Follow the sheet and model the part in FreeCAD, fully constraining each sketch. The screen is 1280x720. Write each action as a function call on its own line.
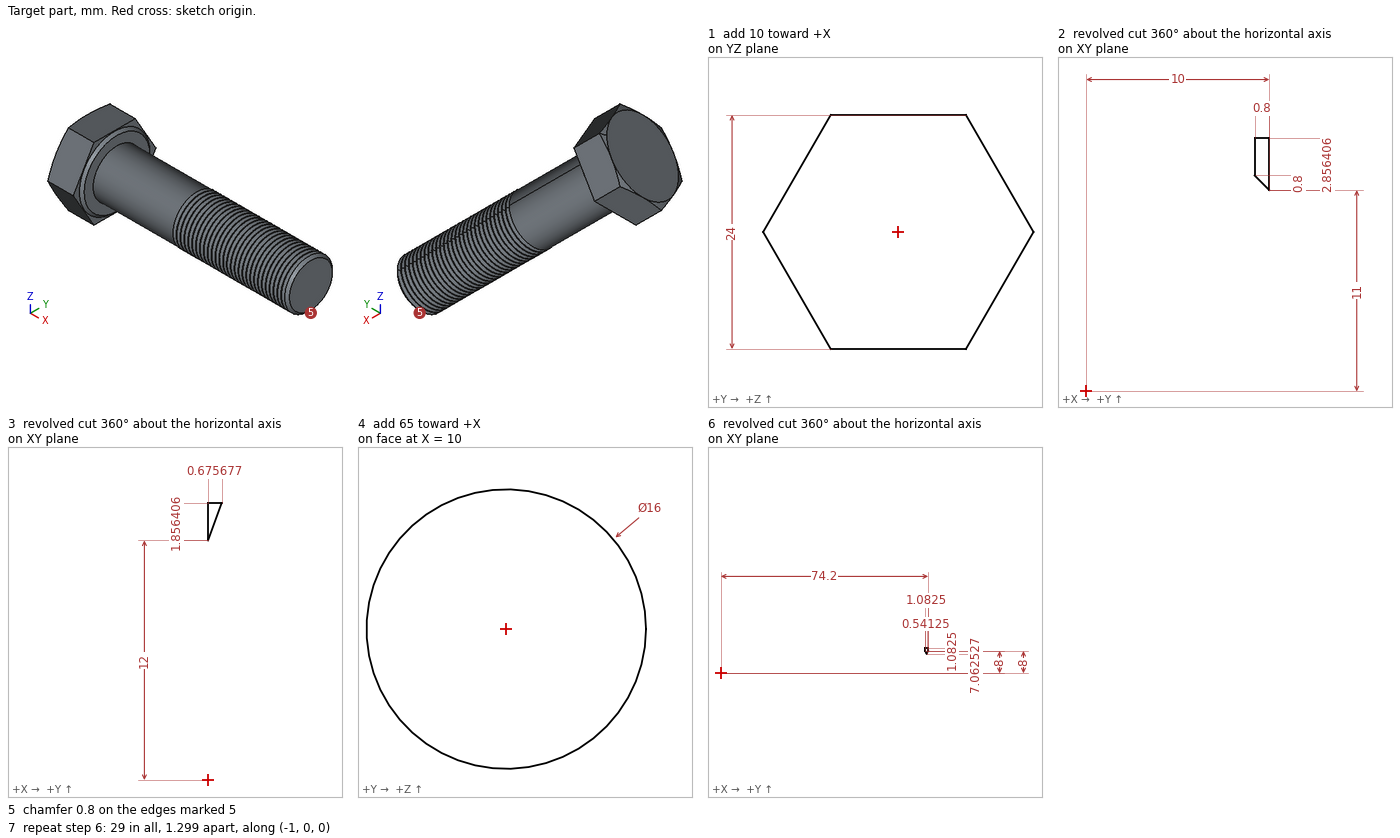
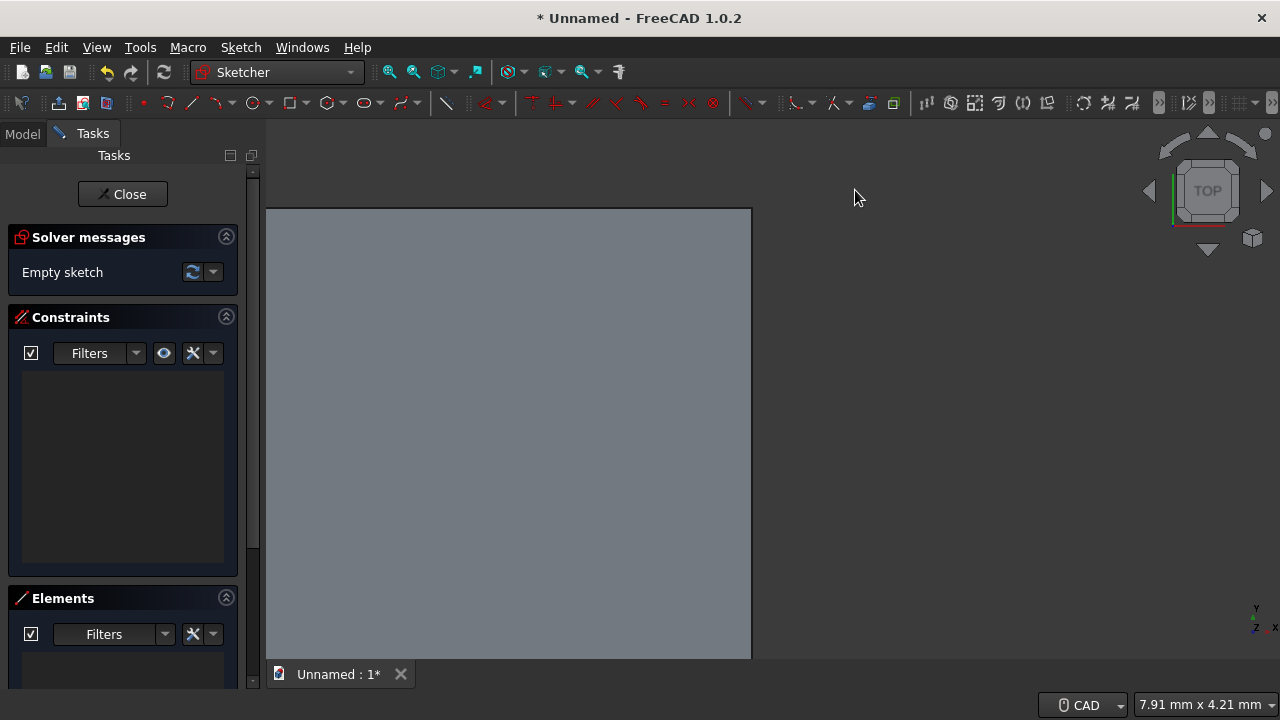
key(g)
key(m)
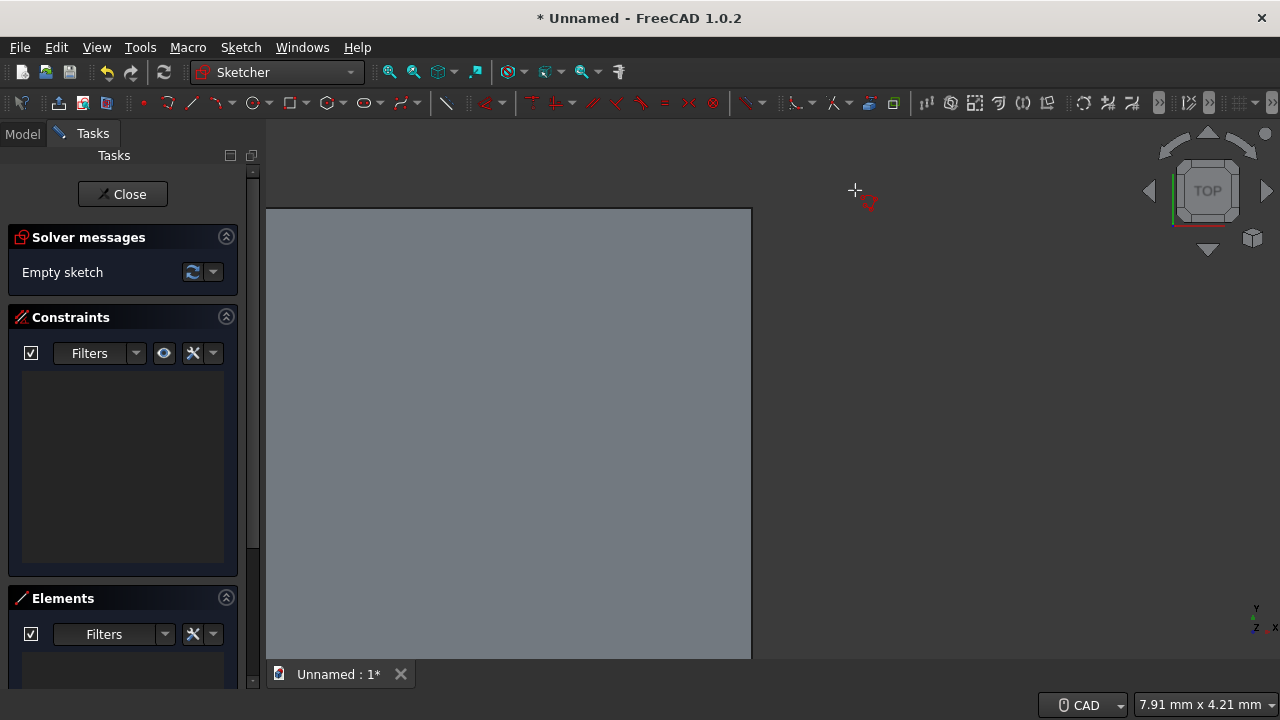
click(752, 574)
click(752, 208)
click(649, 208)
click(649, 472)
click(752, 575)
key(Escape)
key(Escape)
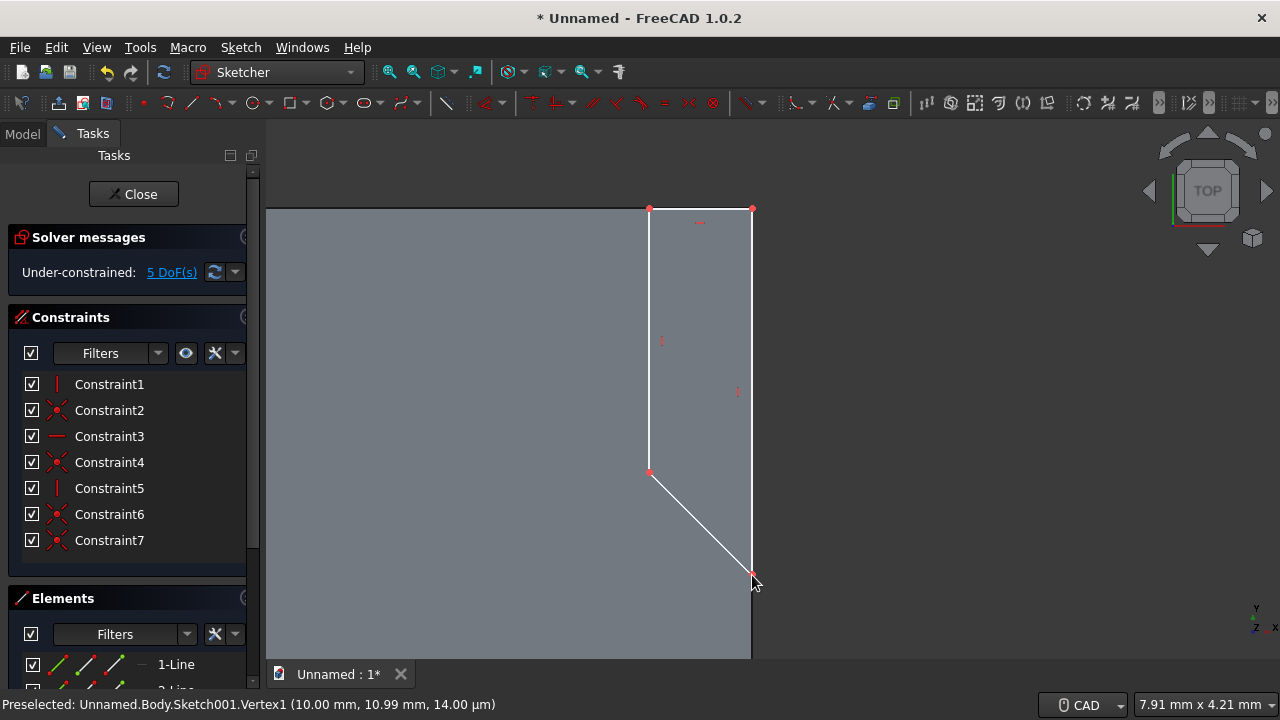
click(486, 104)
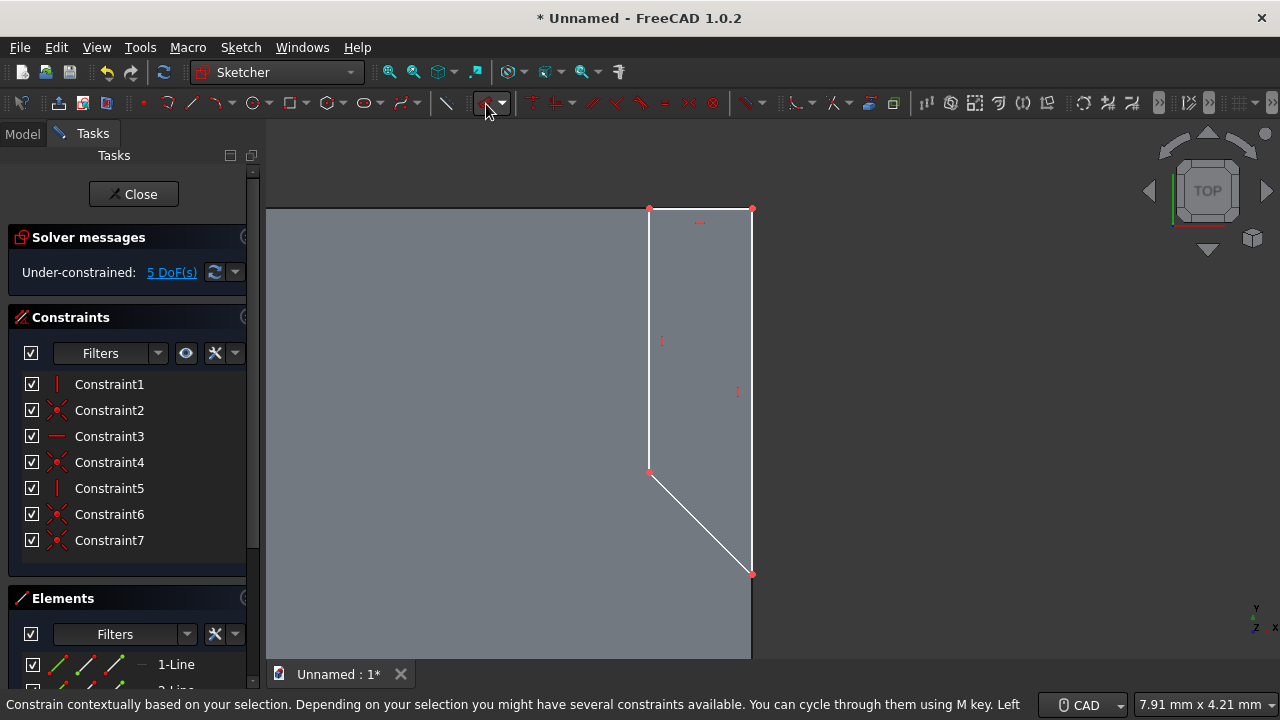
click(721, 209)
click(701, 175)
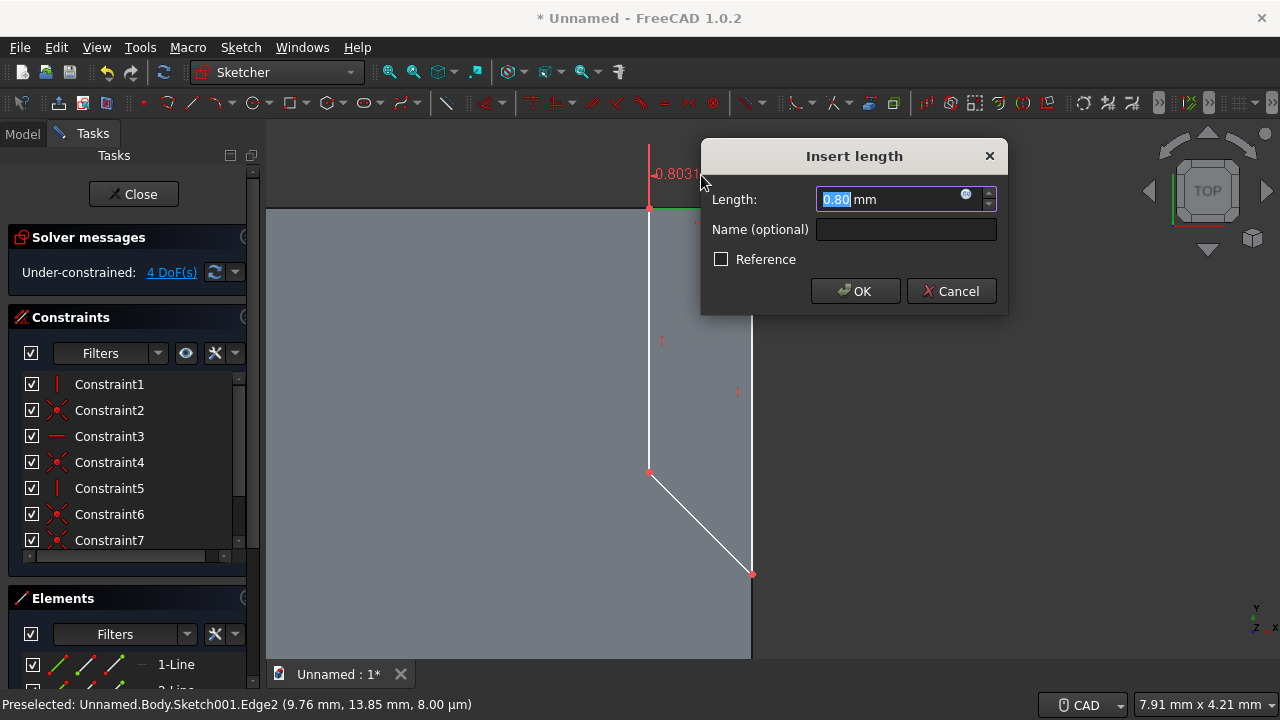
text(0.8)
key(Return)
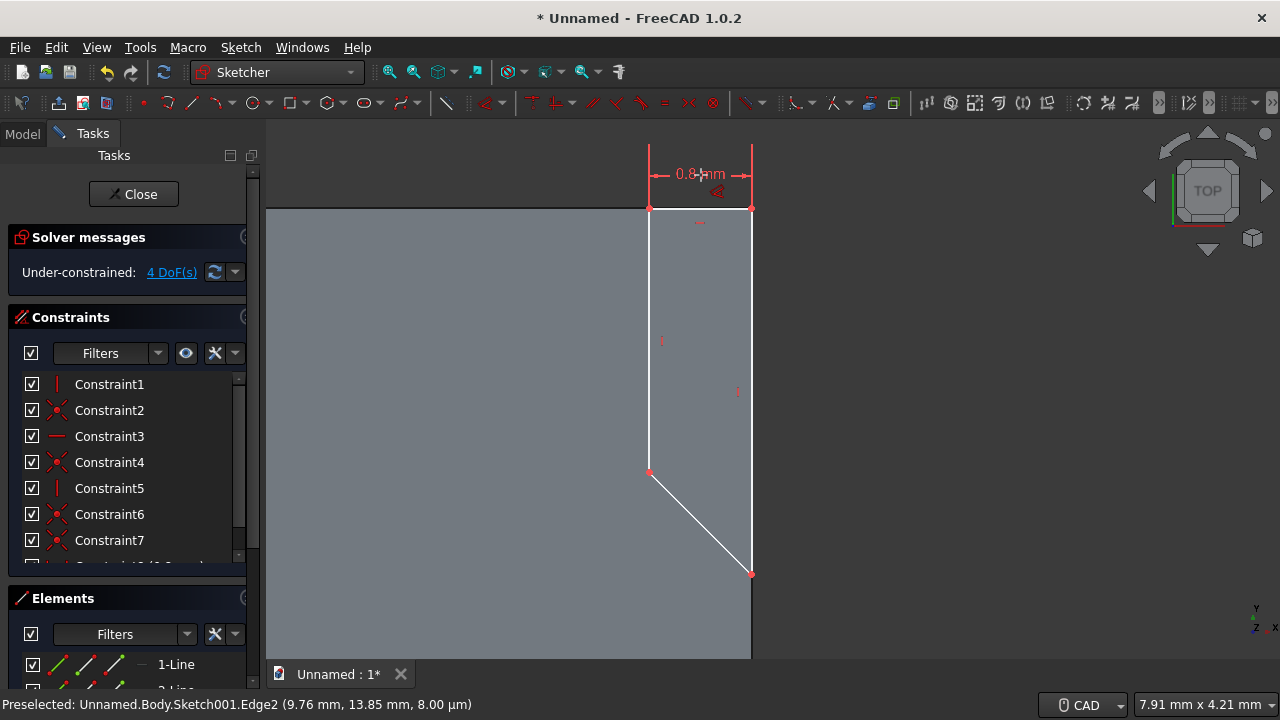
click(752, 575)
click(523, 541)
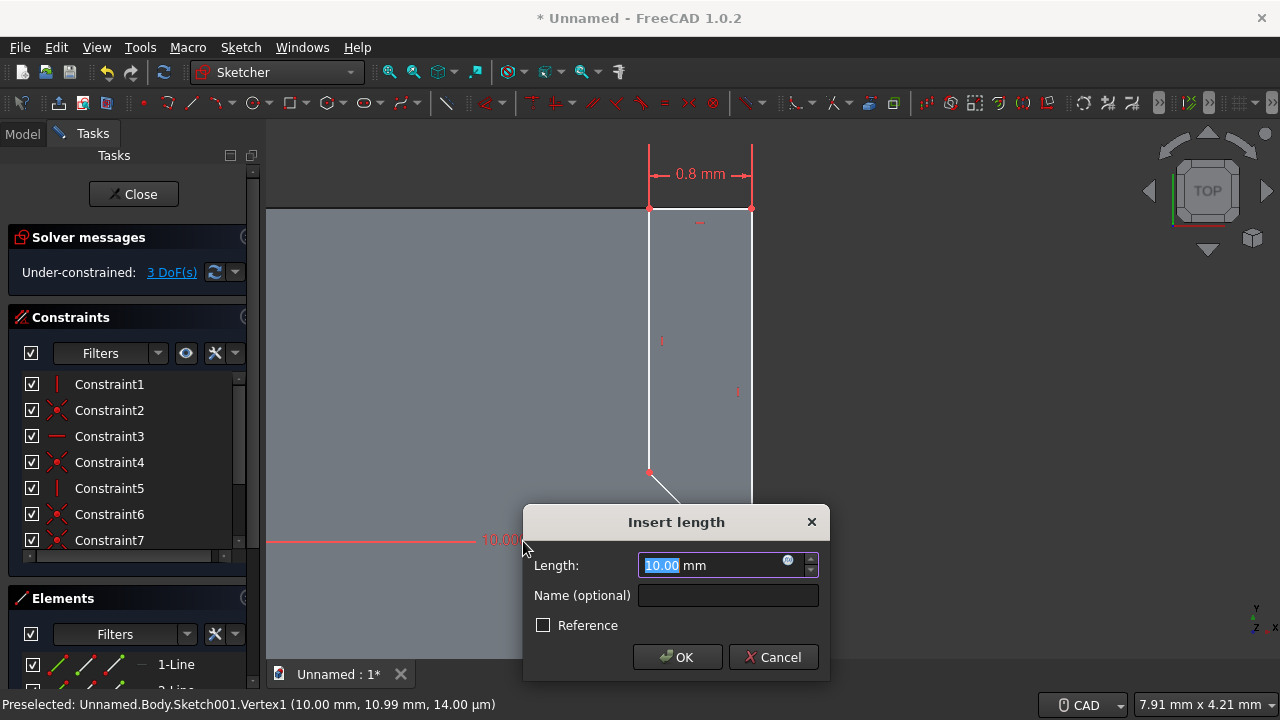
text(10)
key(Return)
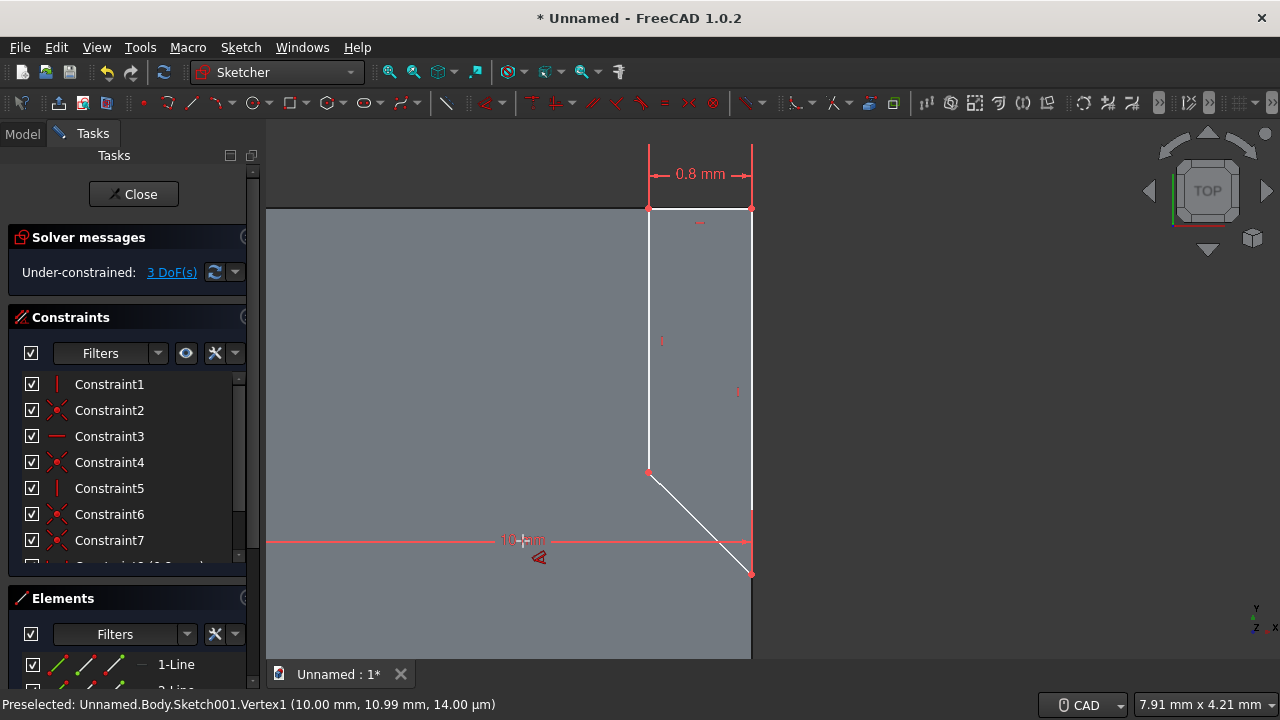
click(752, 575)
click(786, 603)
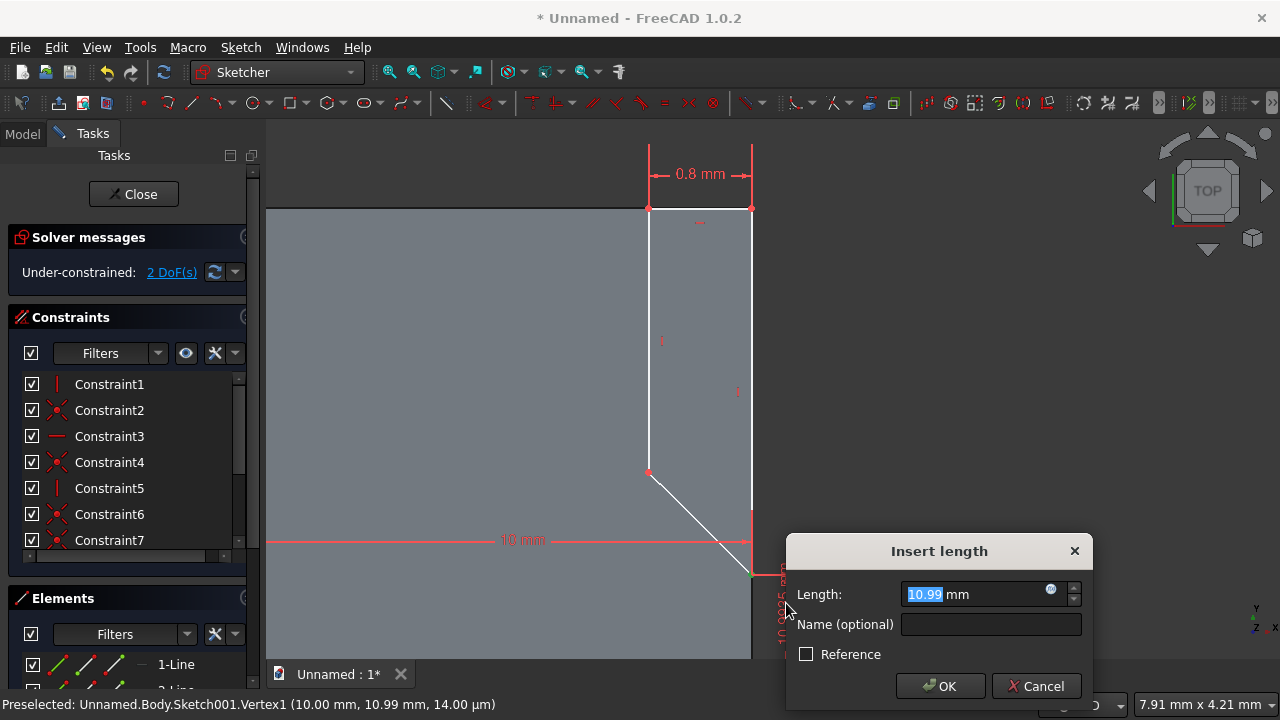
text(11)
key(Return)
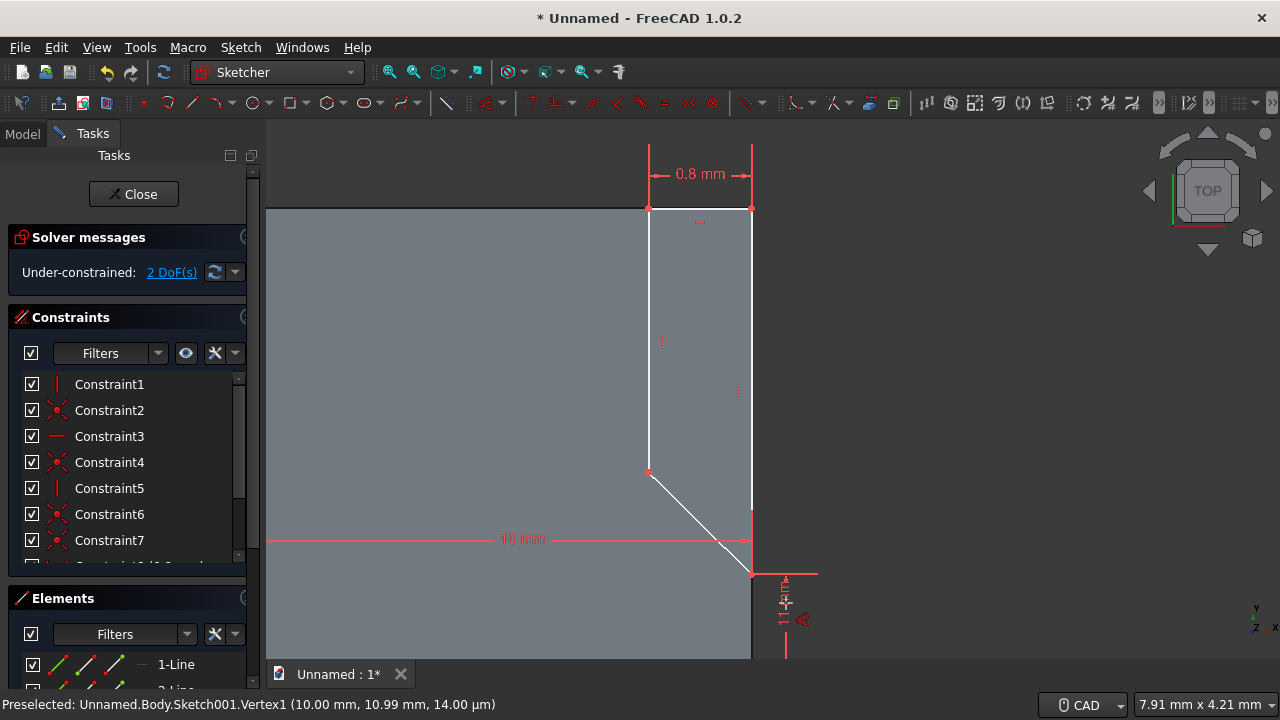
click(680, 503)
click(786, 524)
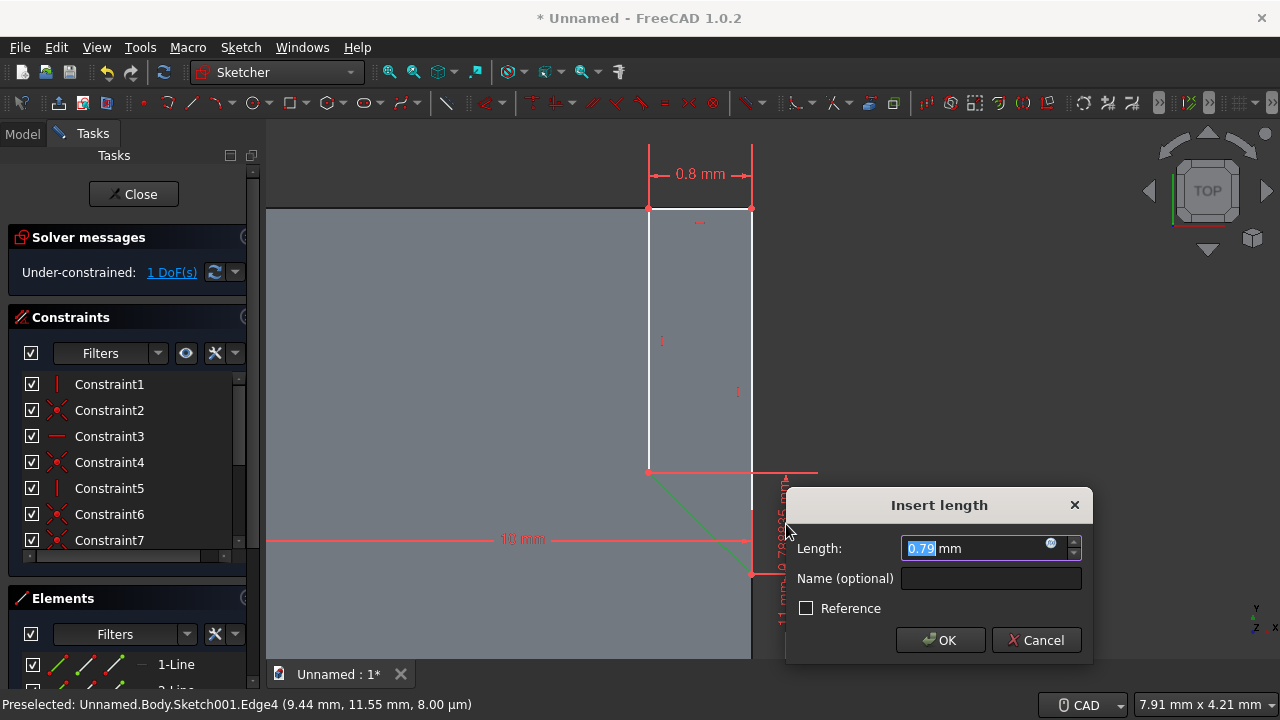
text(0.8)
key(Return)